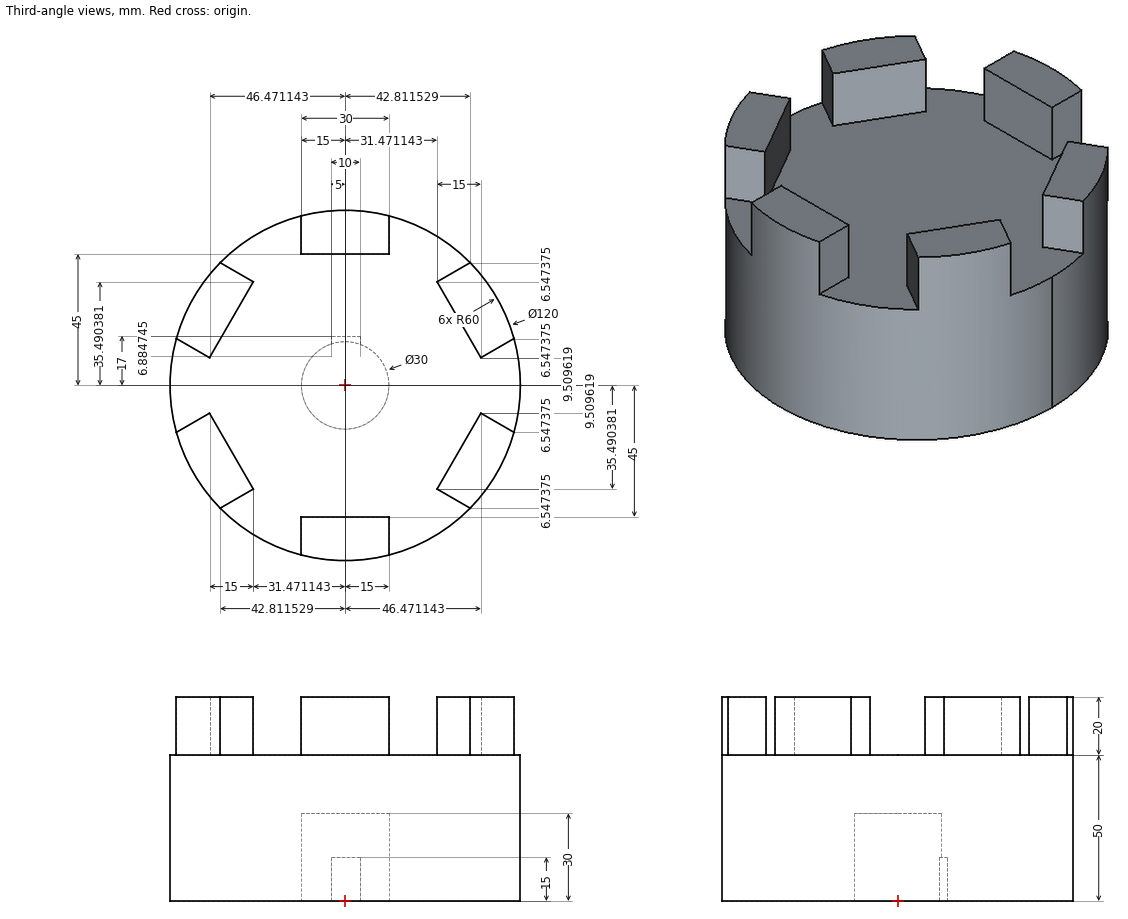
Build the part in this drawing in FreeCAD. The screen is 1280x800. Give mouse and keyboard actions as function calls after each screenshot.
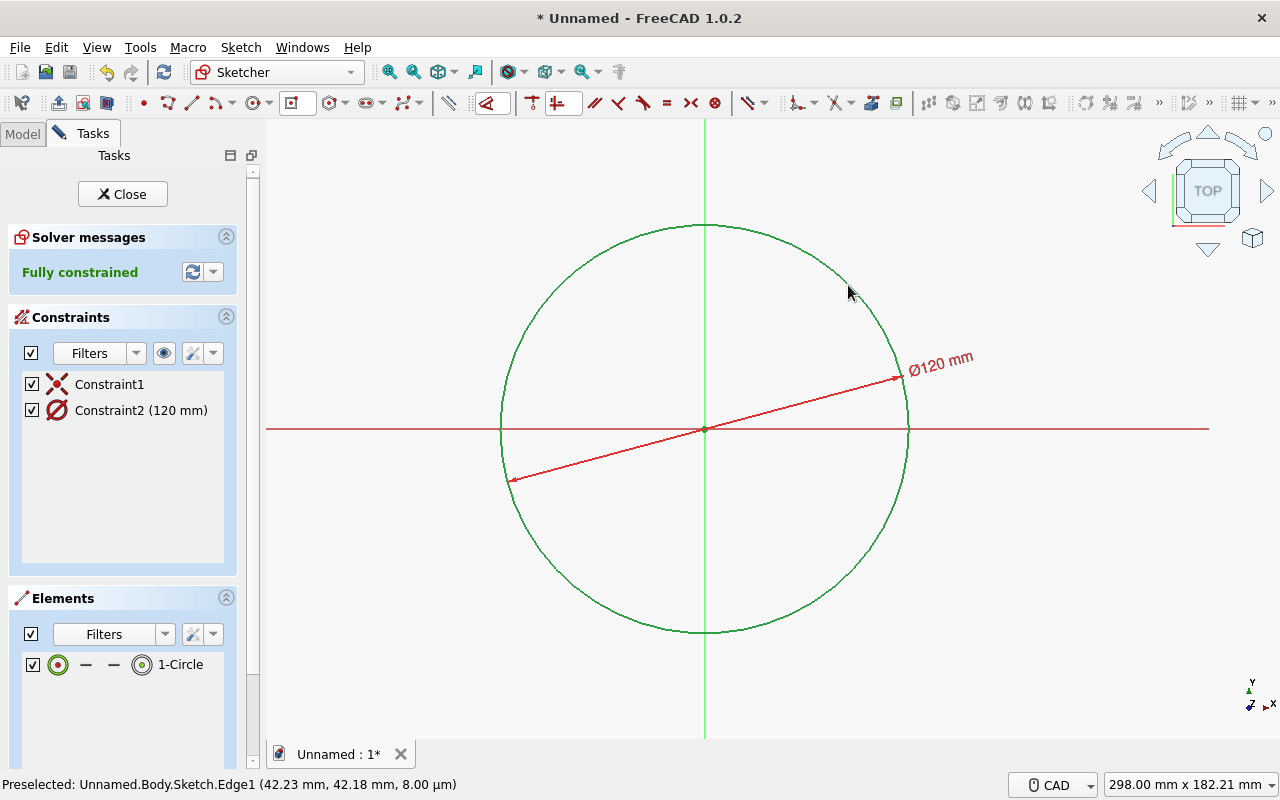
click(123, 194)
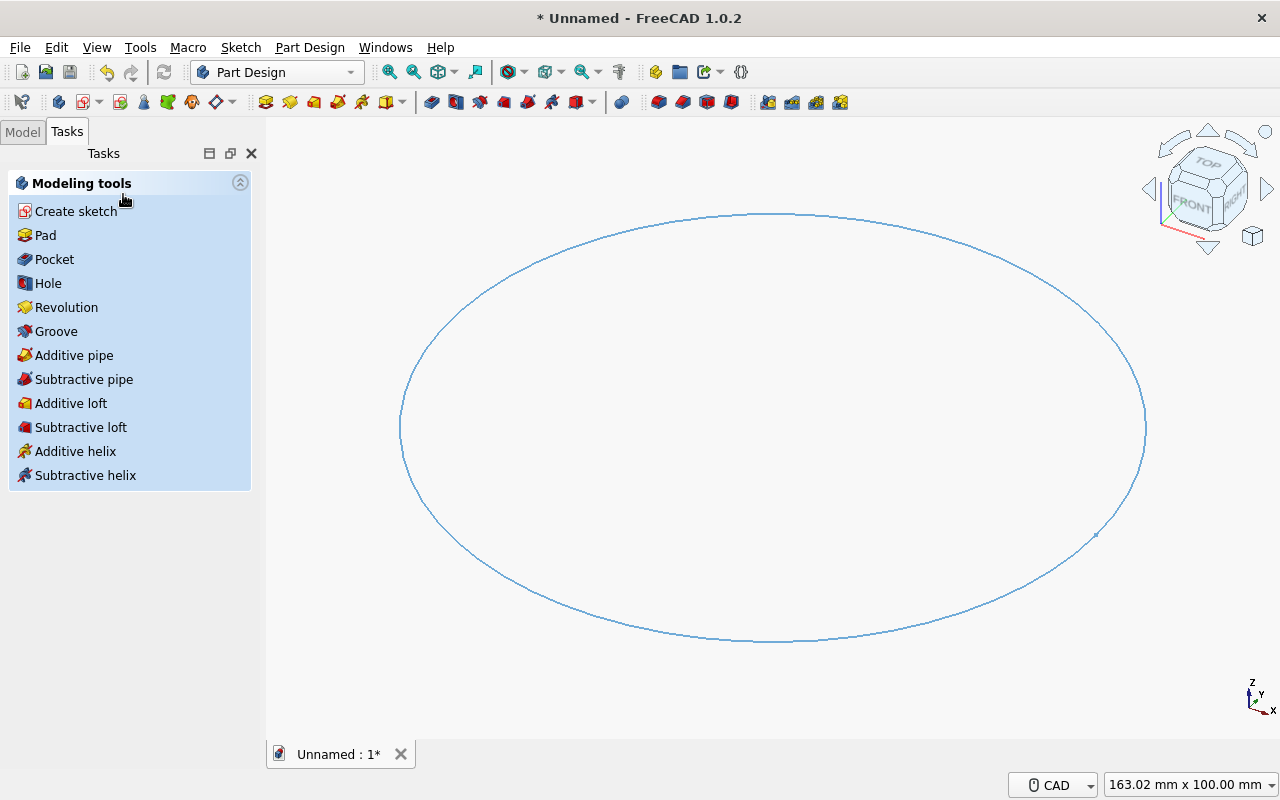
click(266, 102)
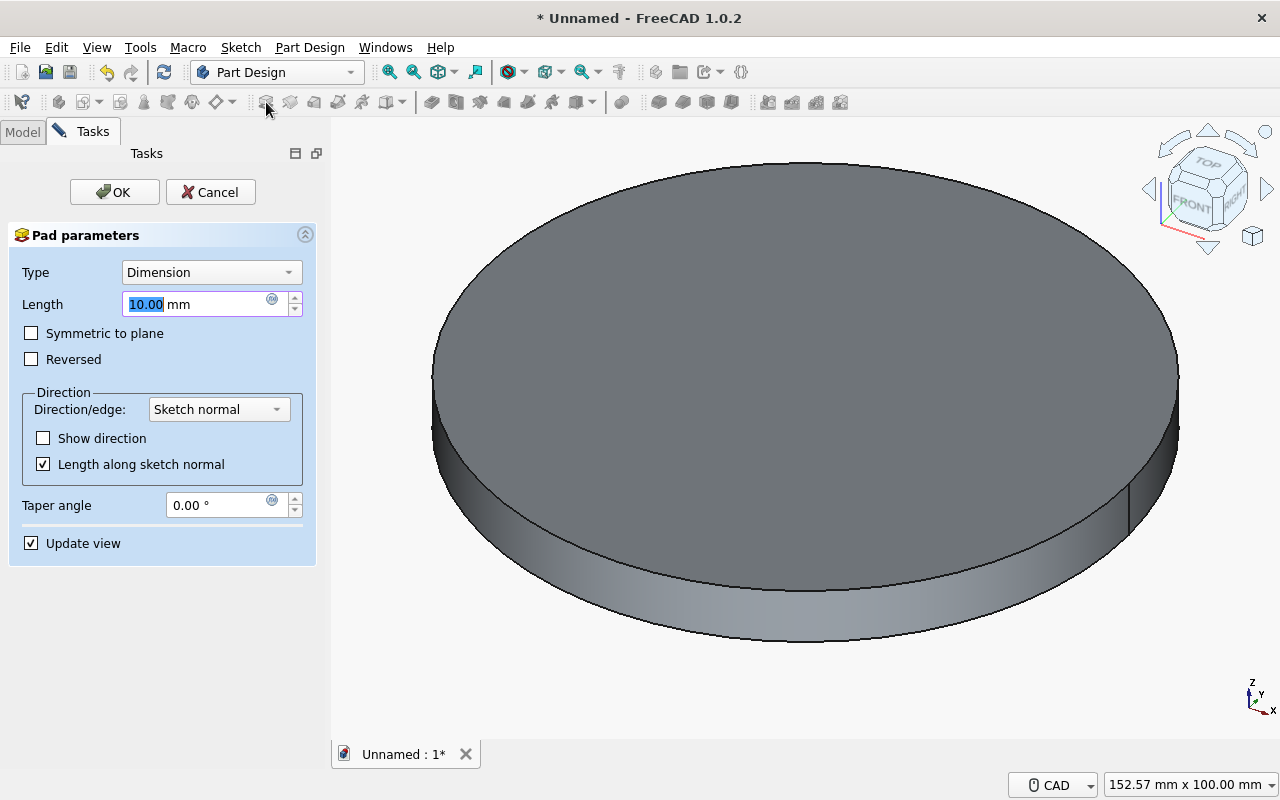
text(50)
key(Tab)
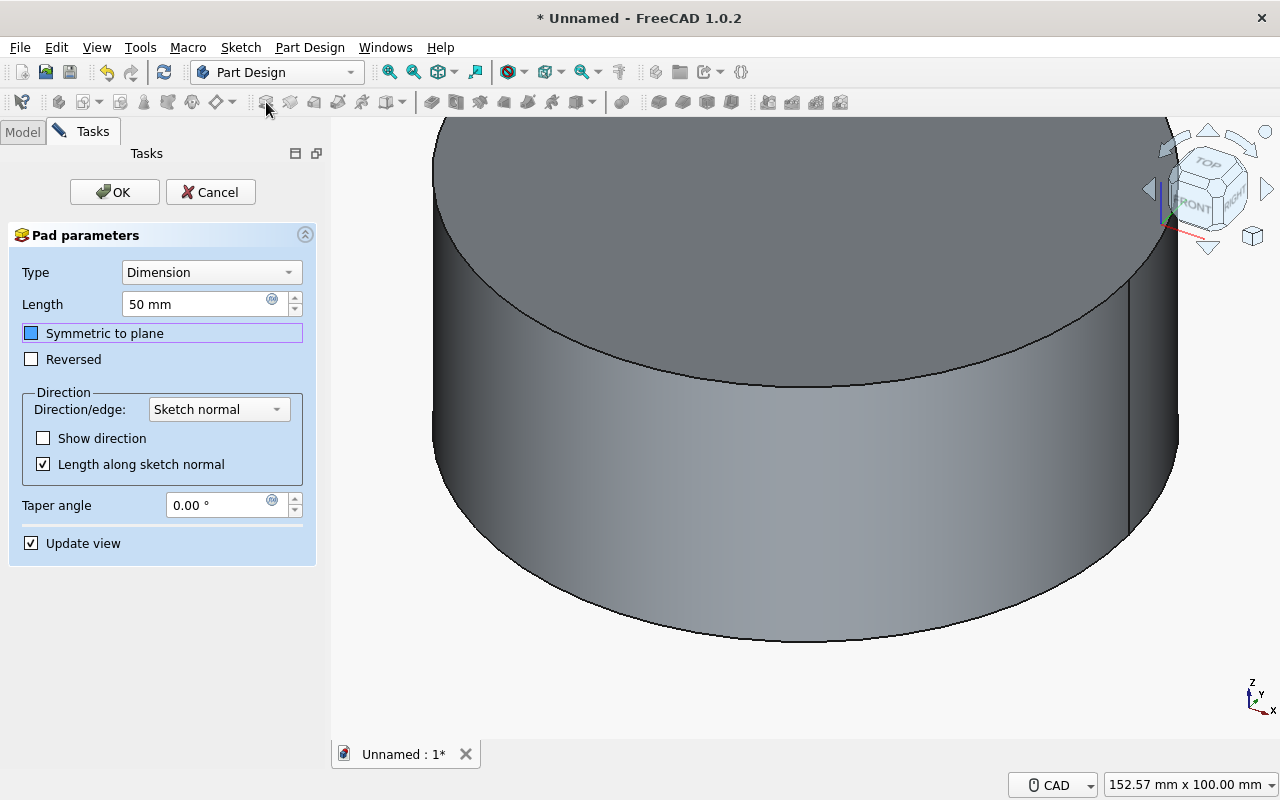
click(115, 192)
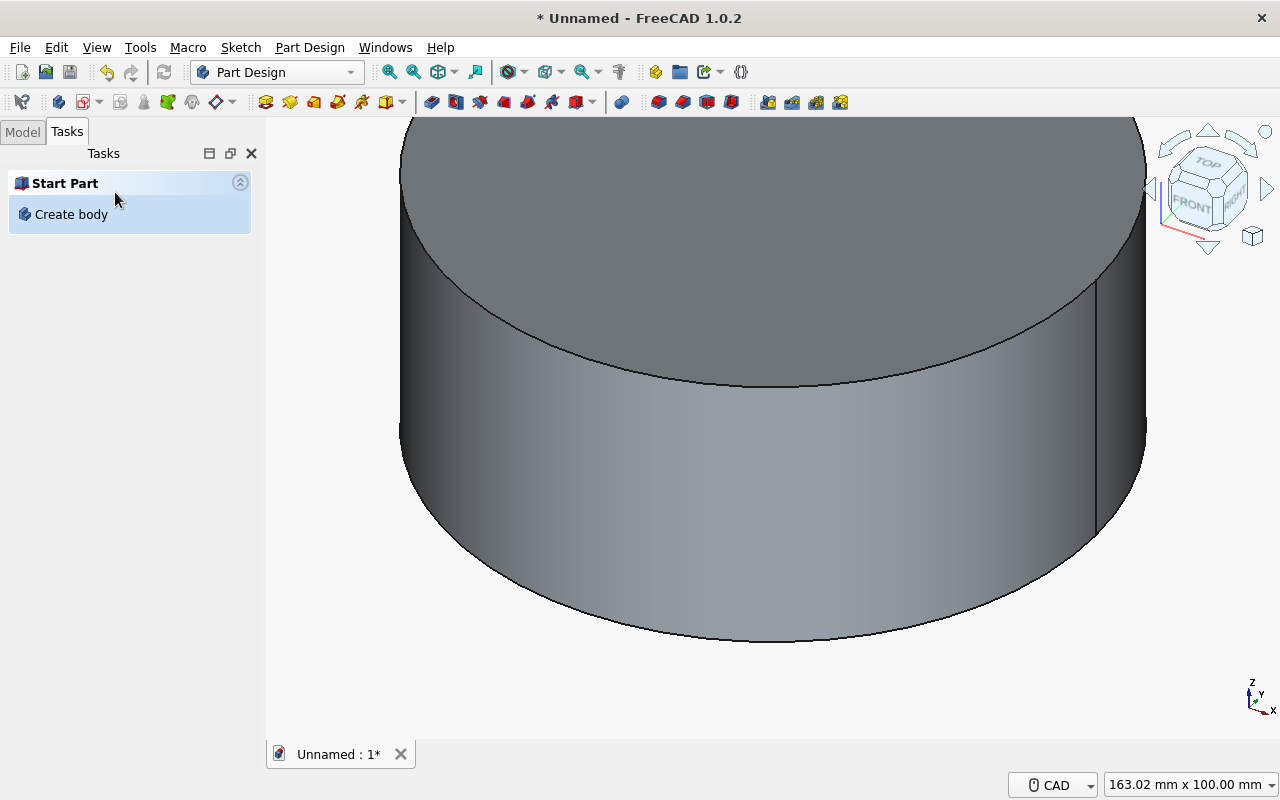
key(v)
key(f)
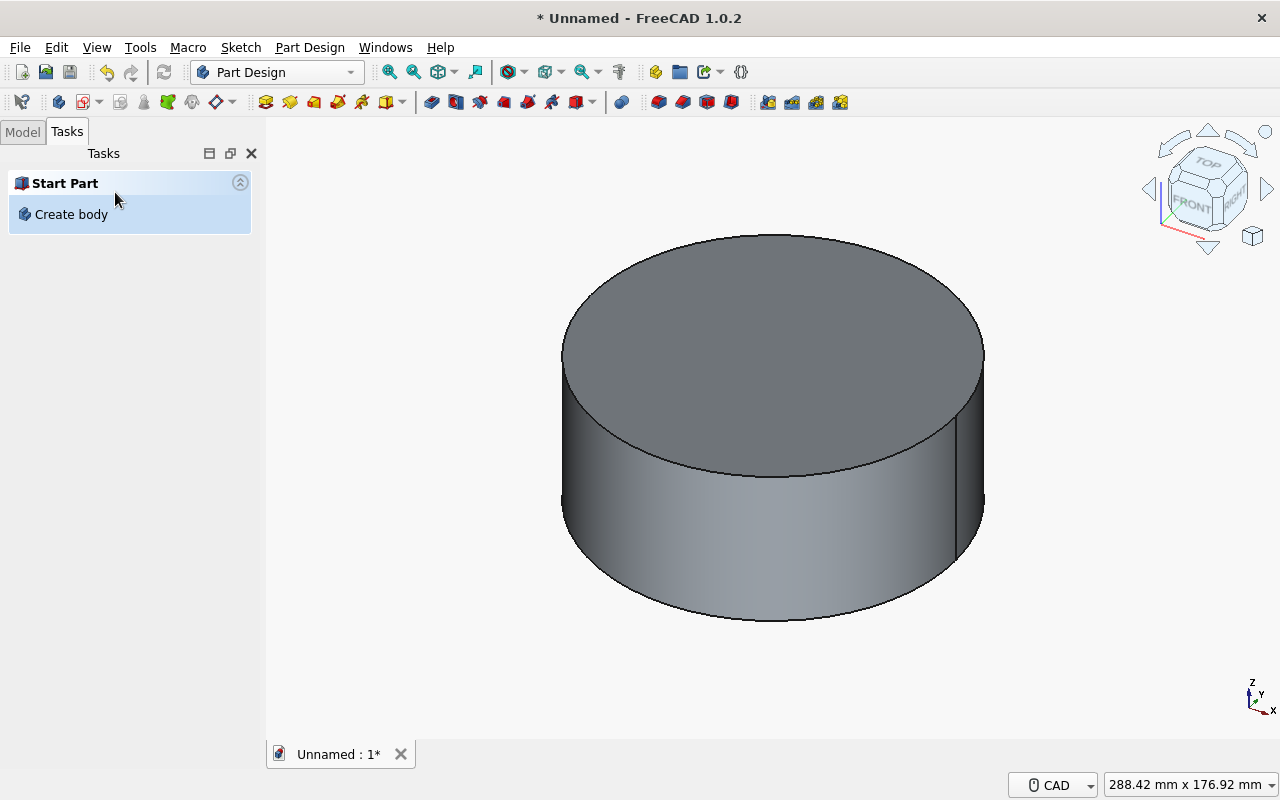
click(84, 102)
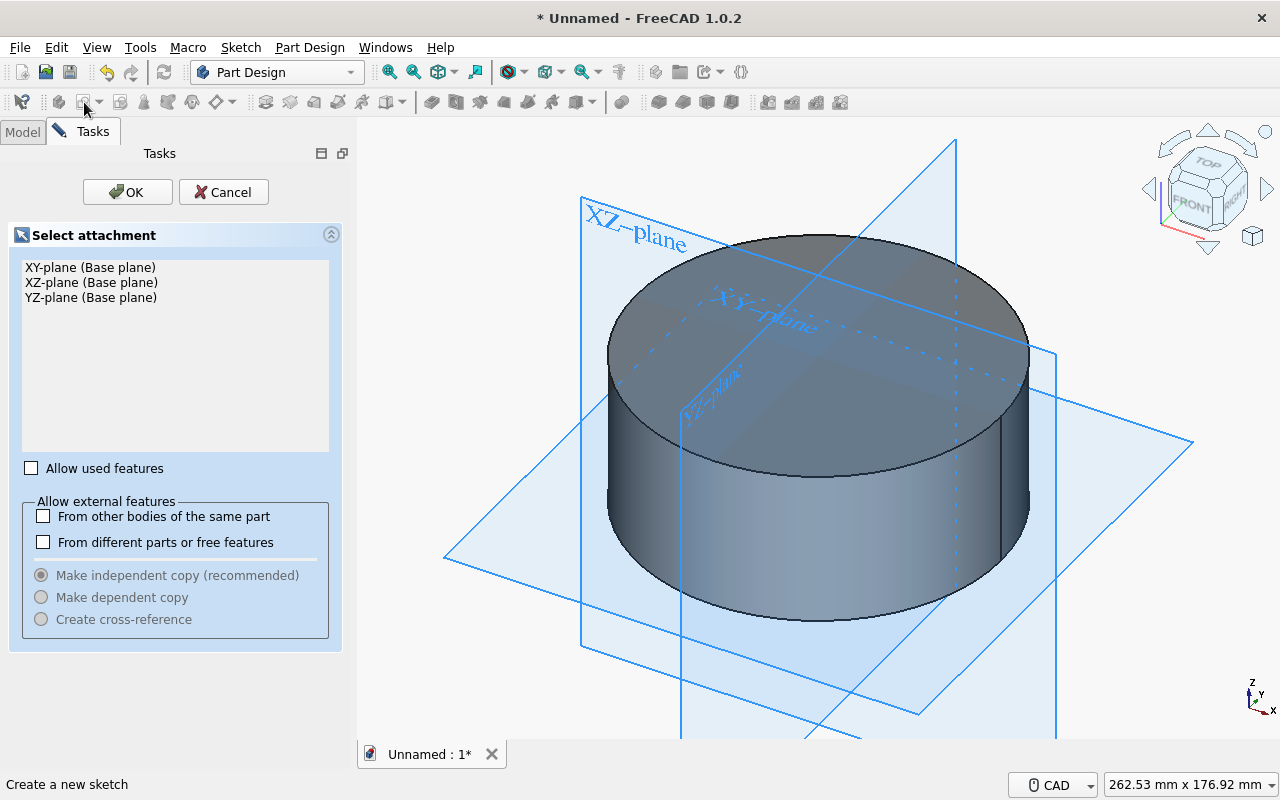
click(82, 268)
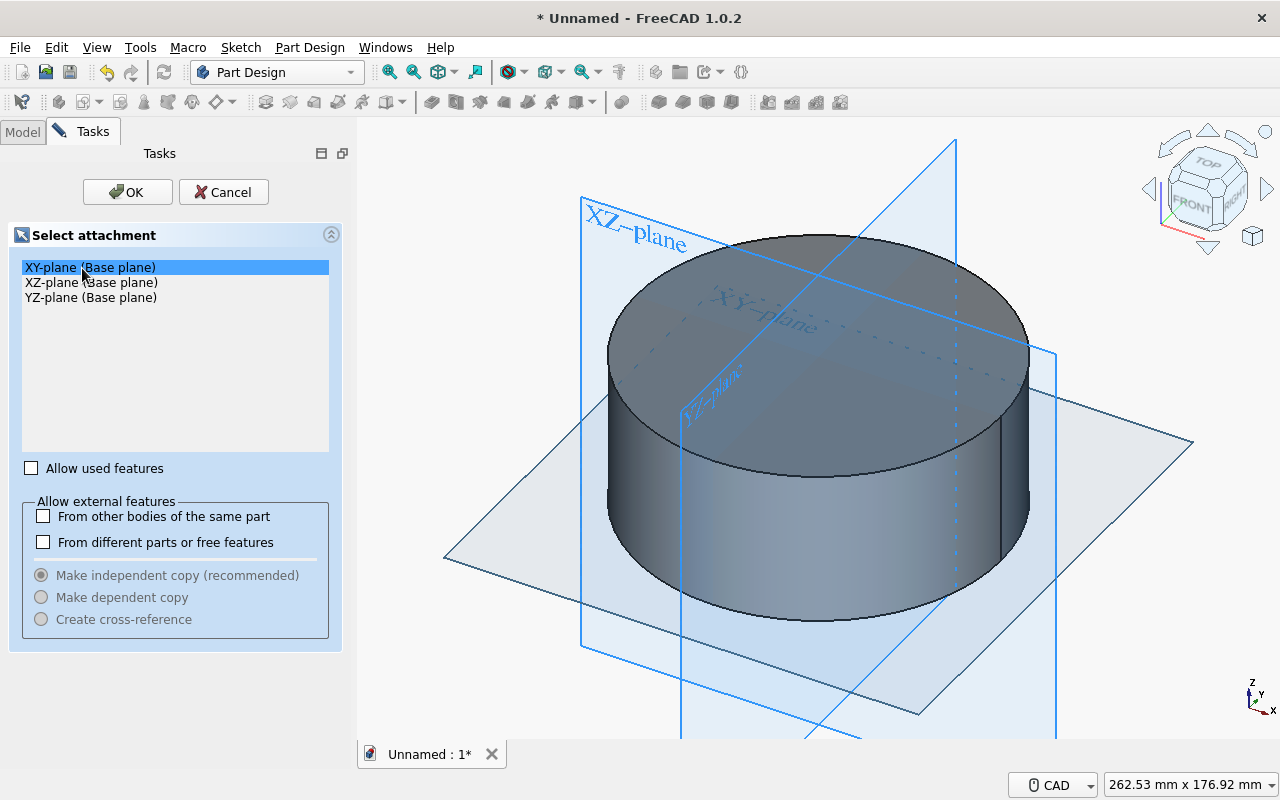
click(128, 192)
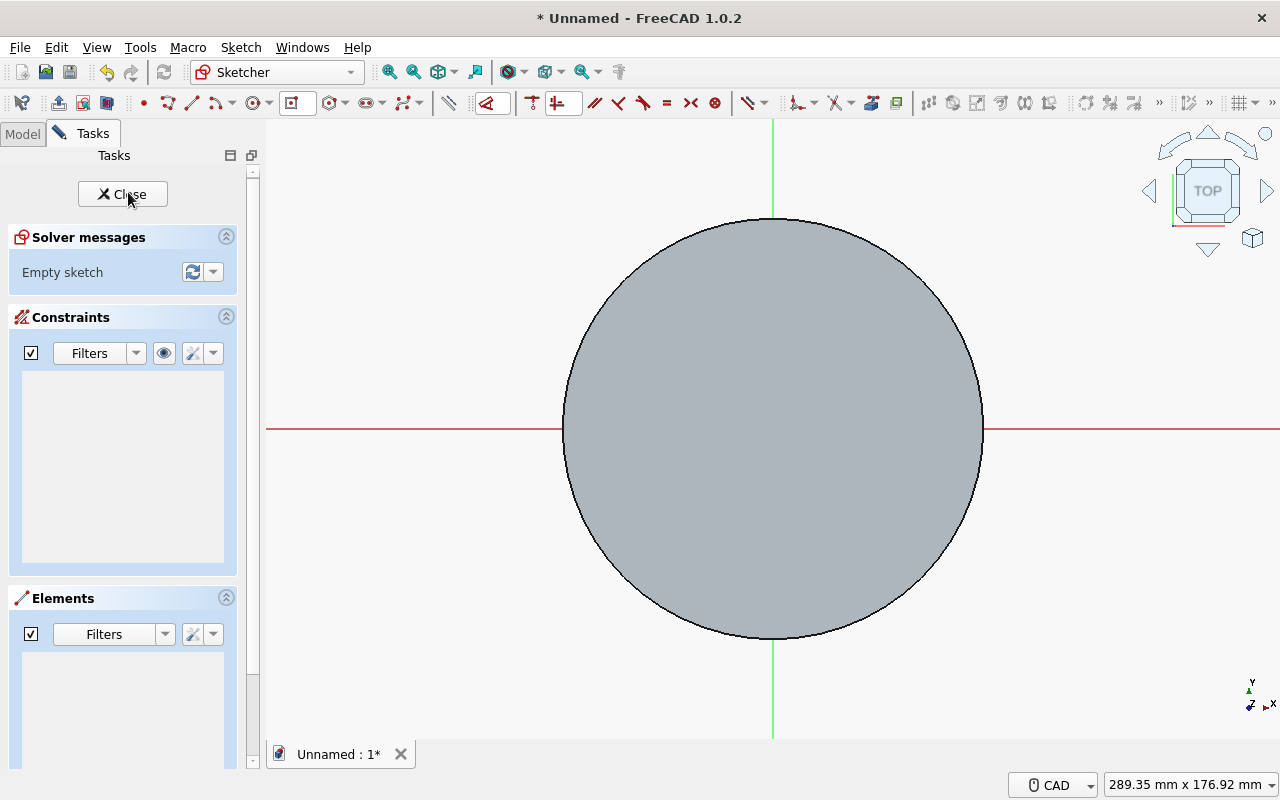
click(108, 104)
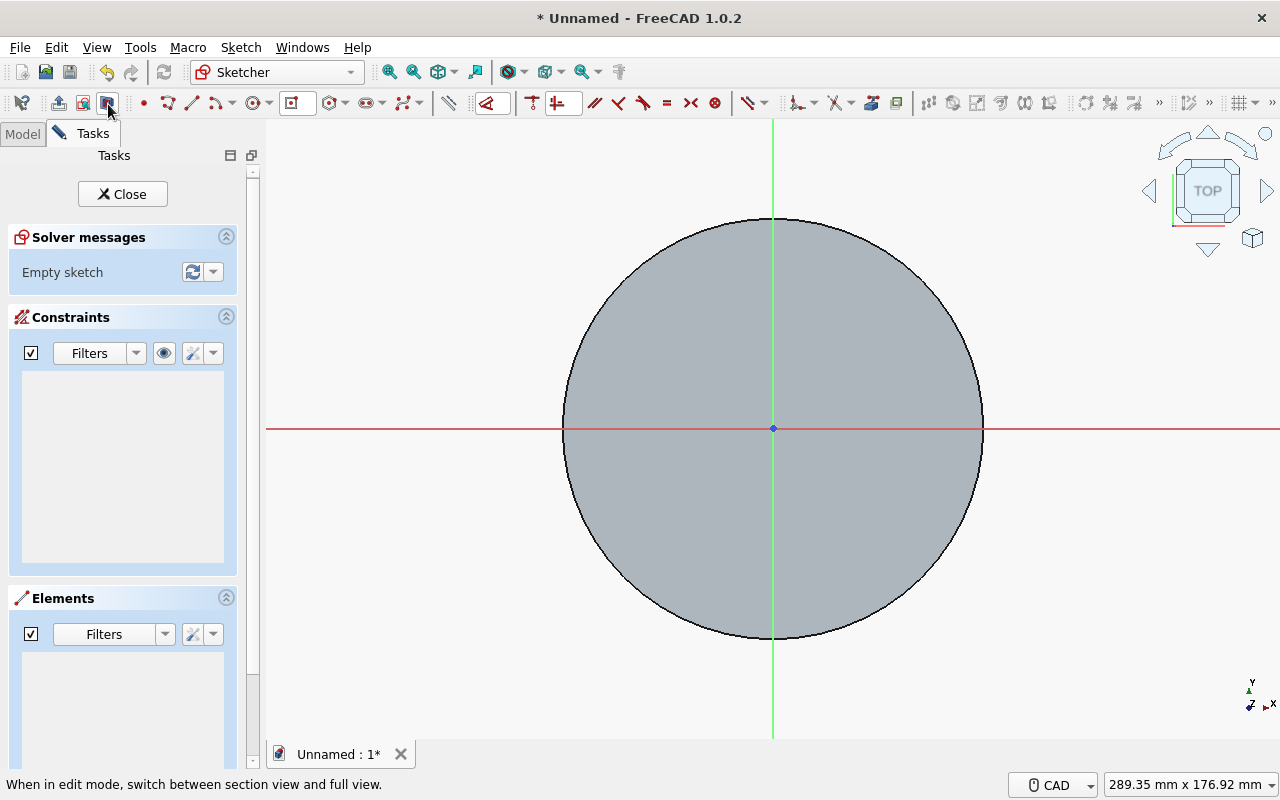
scroll(795, 429, up, 7)